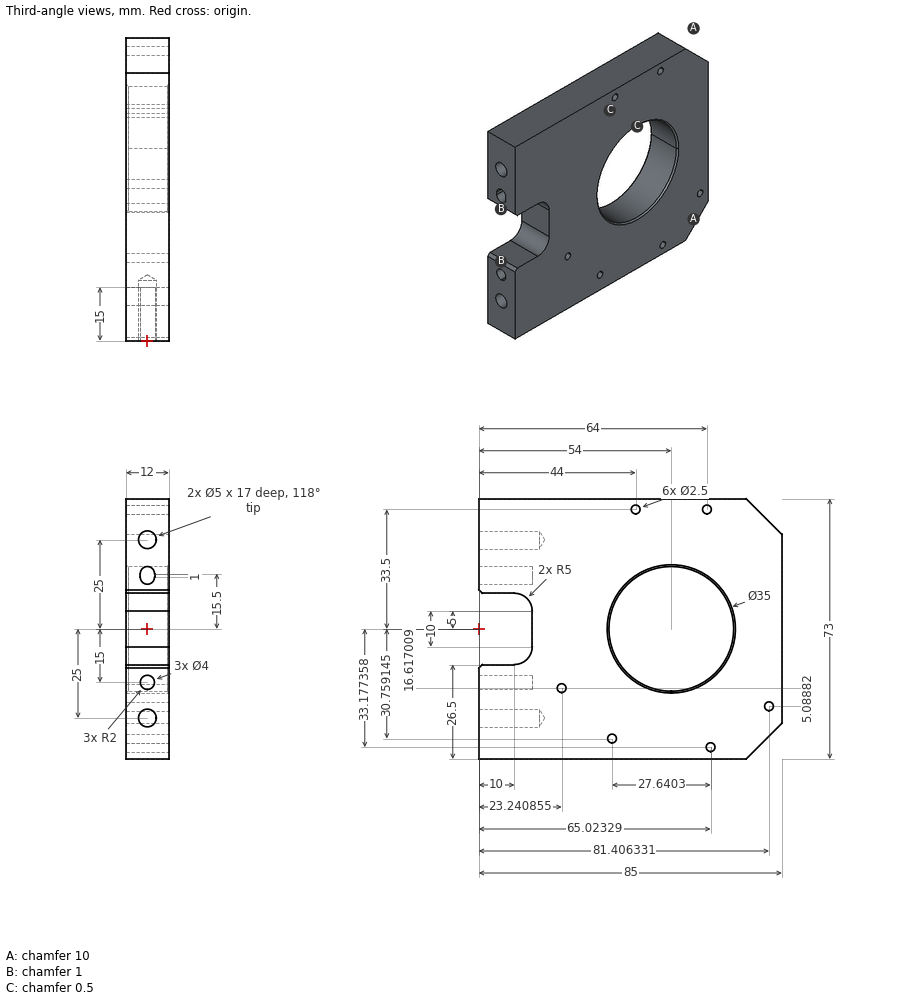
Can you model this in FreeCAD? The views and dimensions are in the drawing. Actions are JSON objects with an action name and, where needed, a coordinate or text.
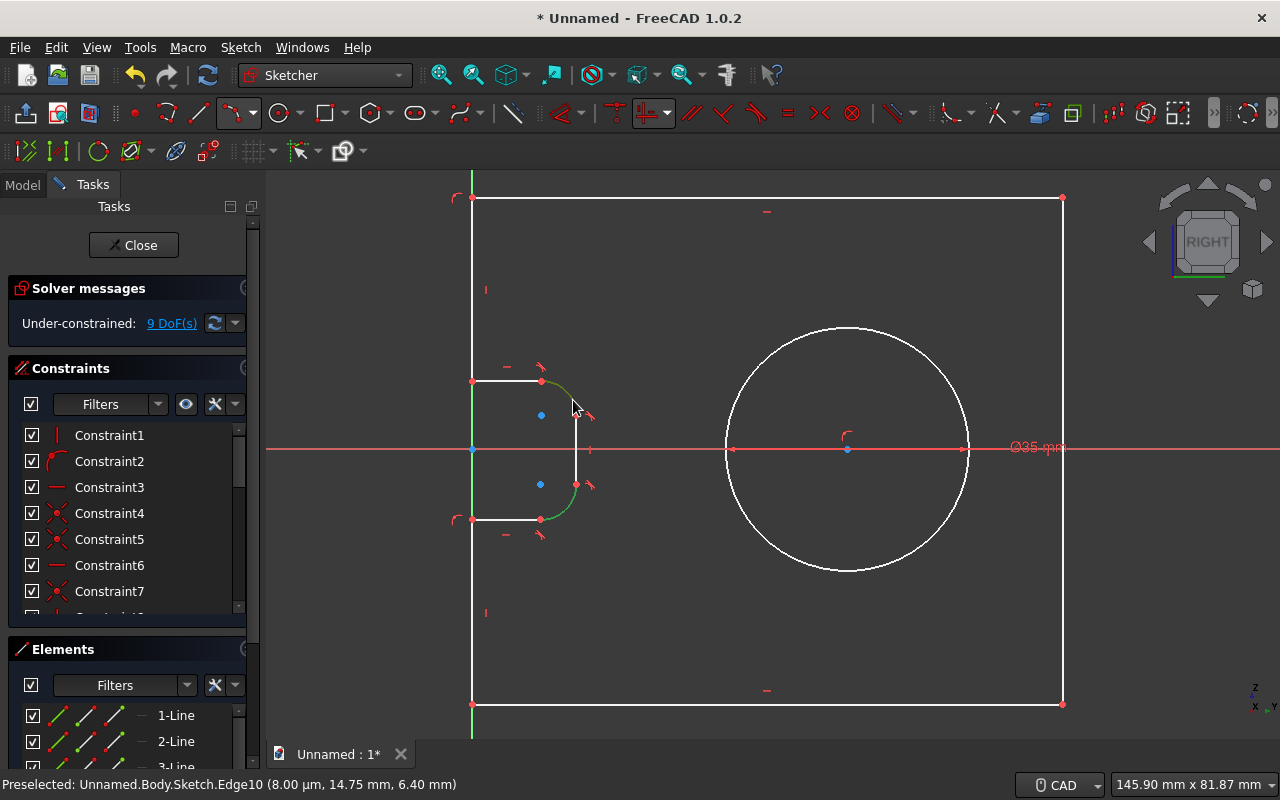
{"action": "left_click", "coordinate": [788, 114]}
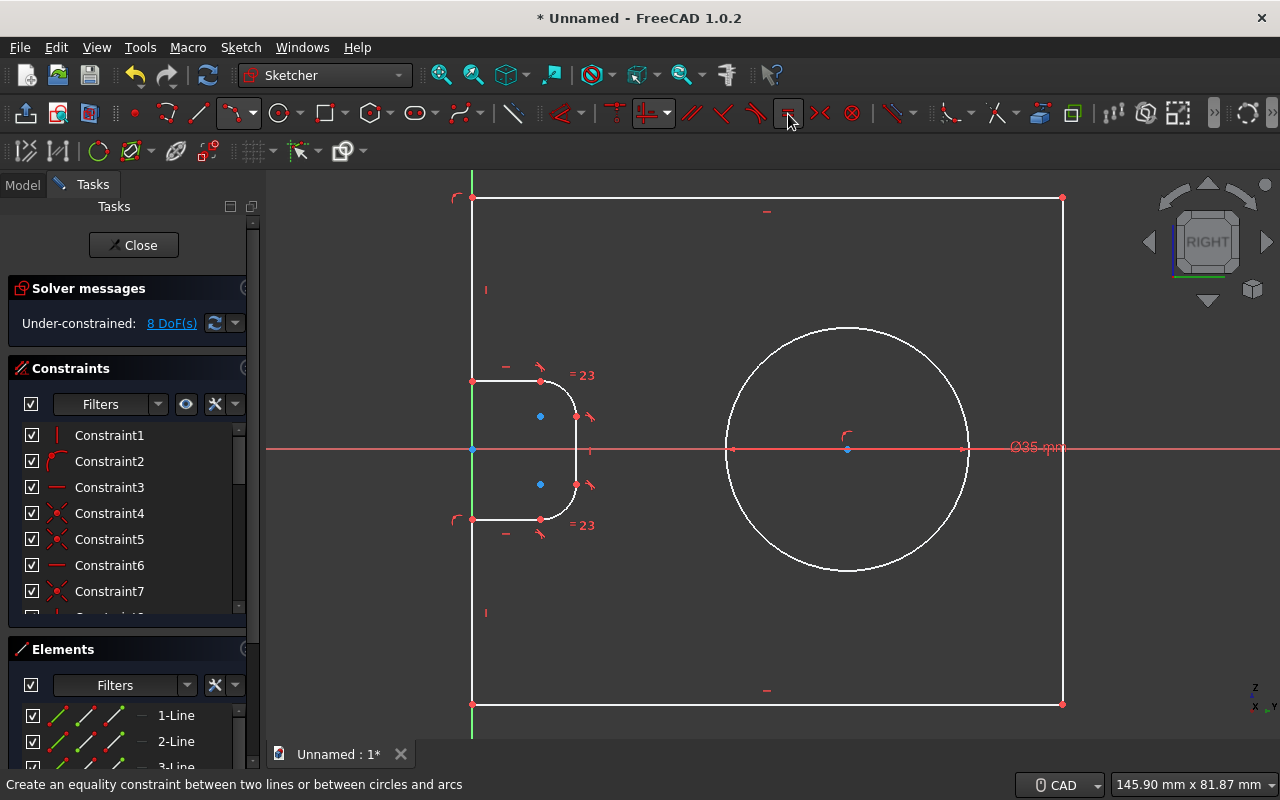
{"action": "left_click", "coordinate": [560, 114]}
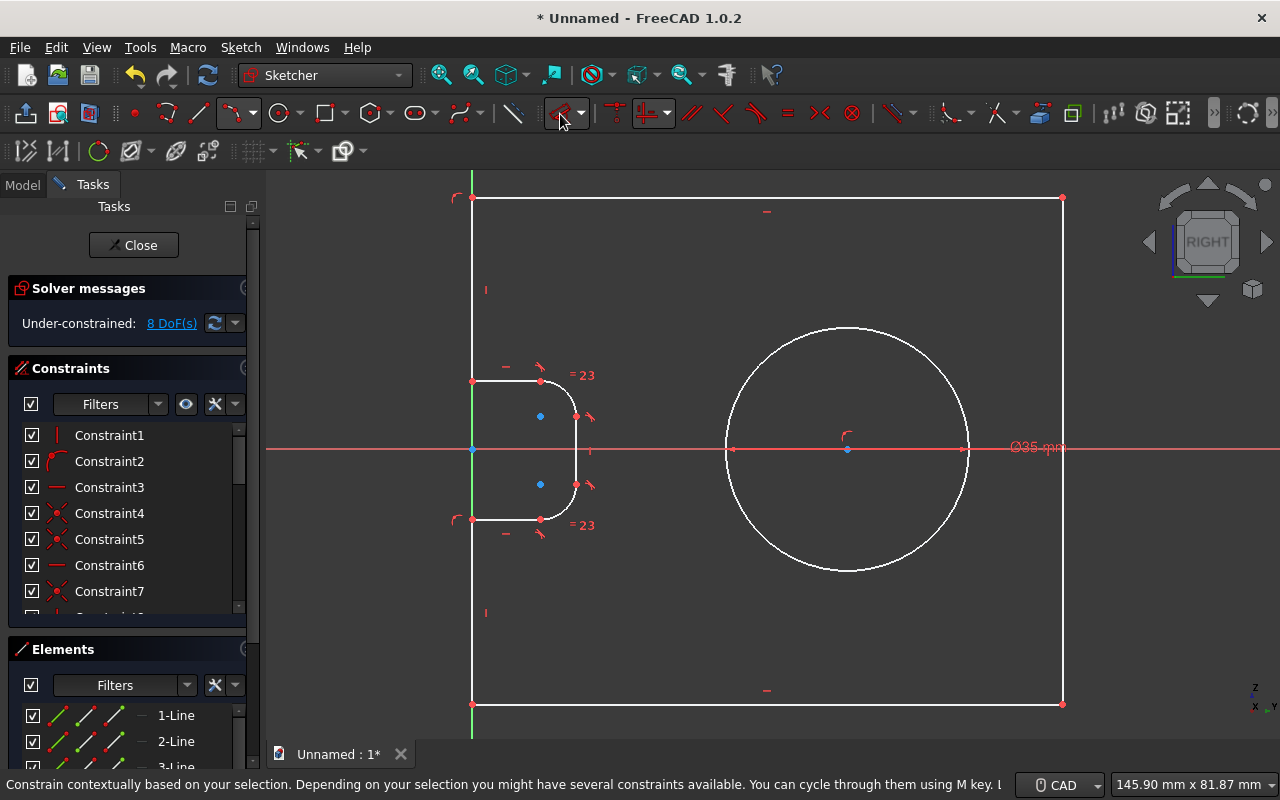
{"action": "left_click", "coordinate": [557, 516]}
{"action": "left_click", "coordinate": [572, 544]}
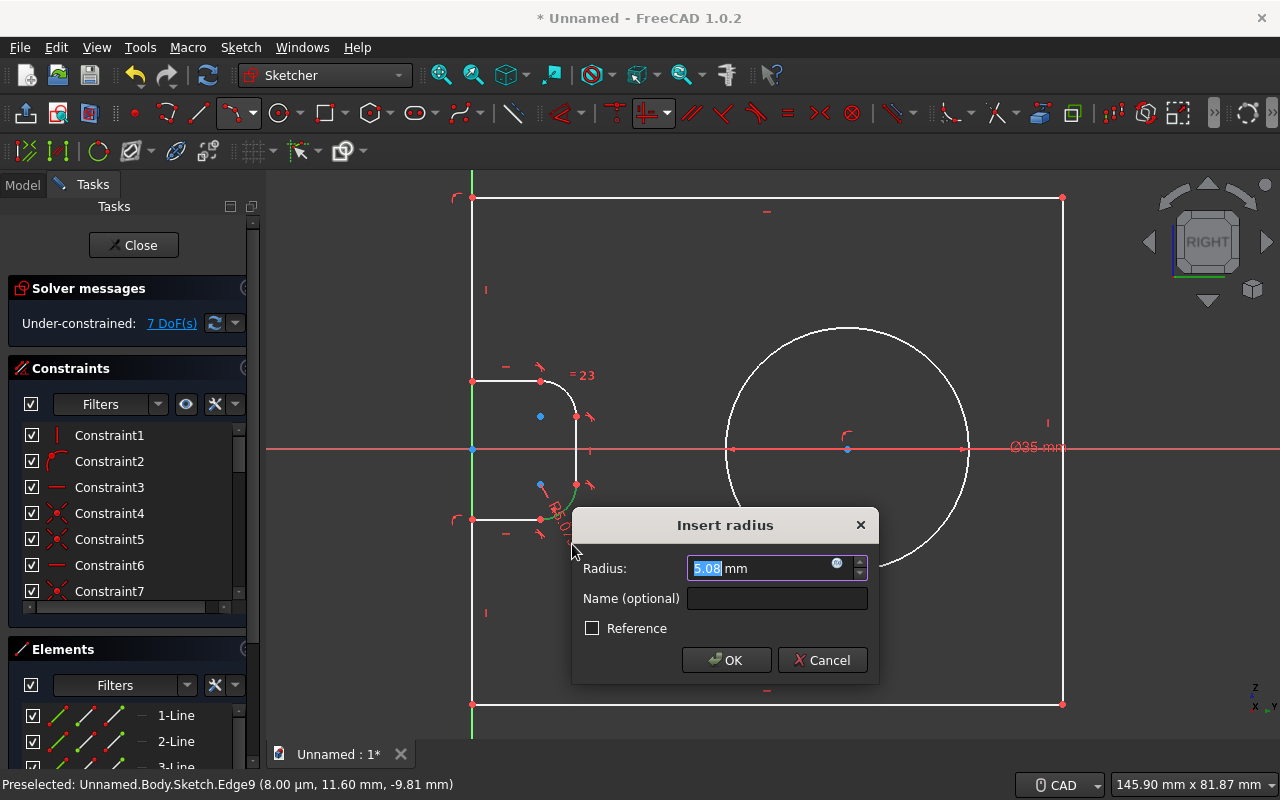
{"action": "type", "text": "5"}
{"action": "key", "text": "Return"}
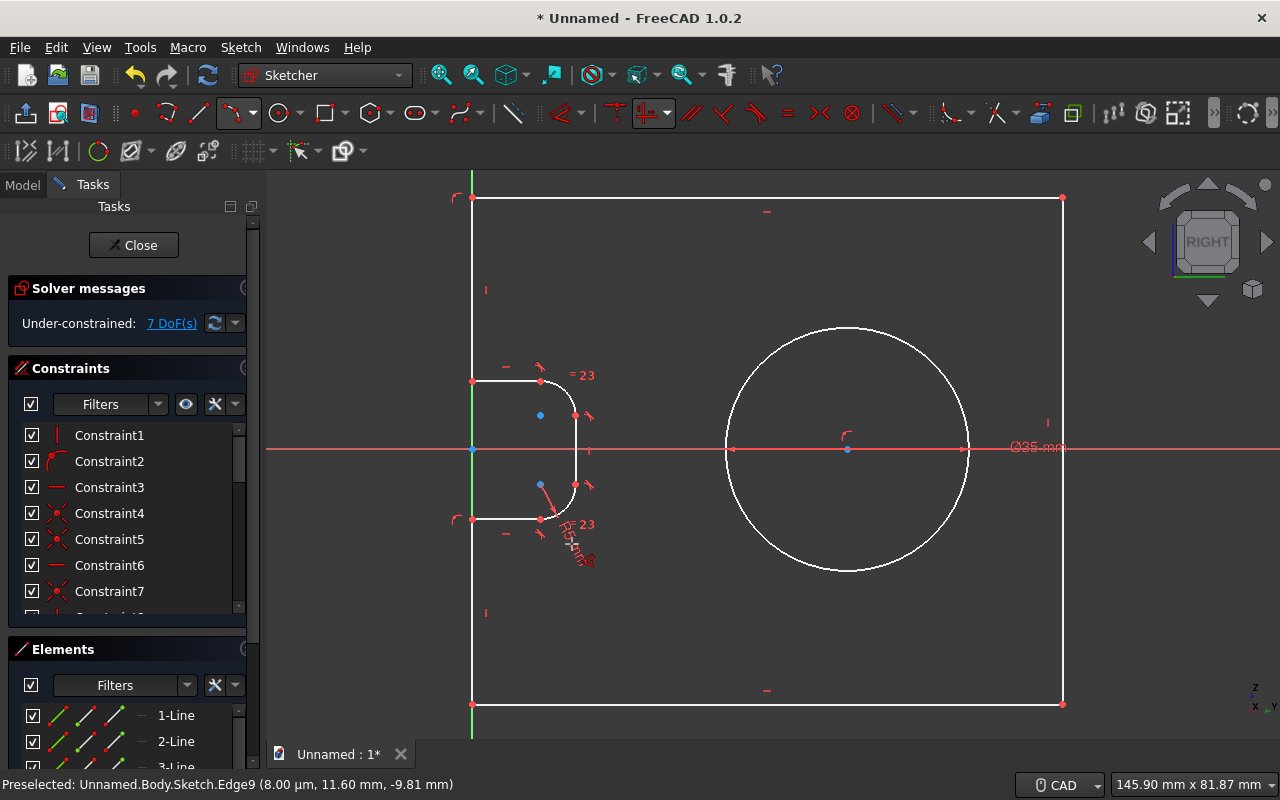
{"action": "left_click", "coordinate": [576, 436]}
{"action": "left_click", "coordinate": [542, 434]}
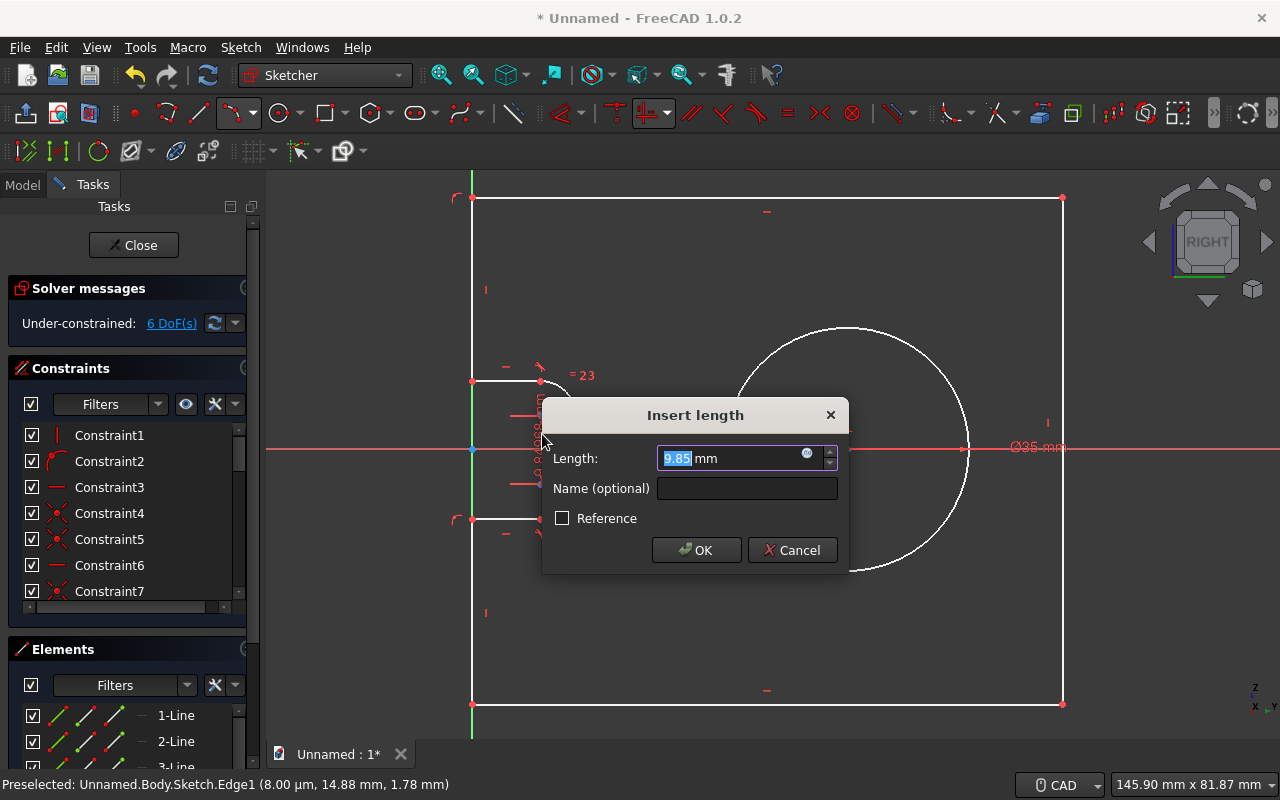
{"action": "type", "text": "10"}
{"action": "key", "text": "Return"}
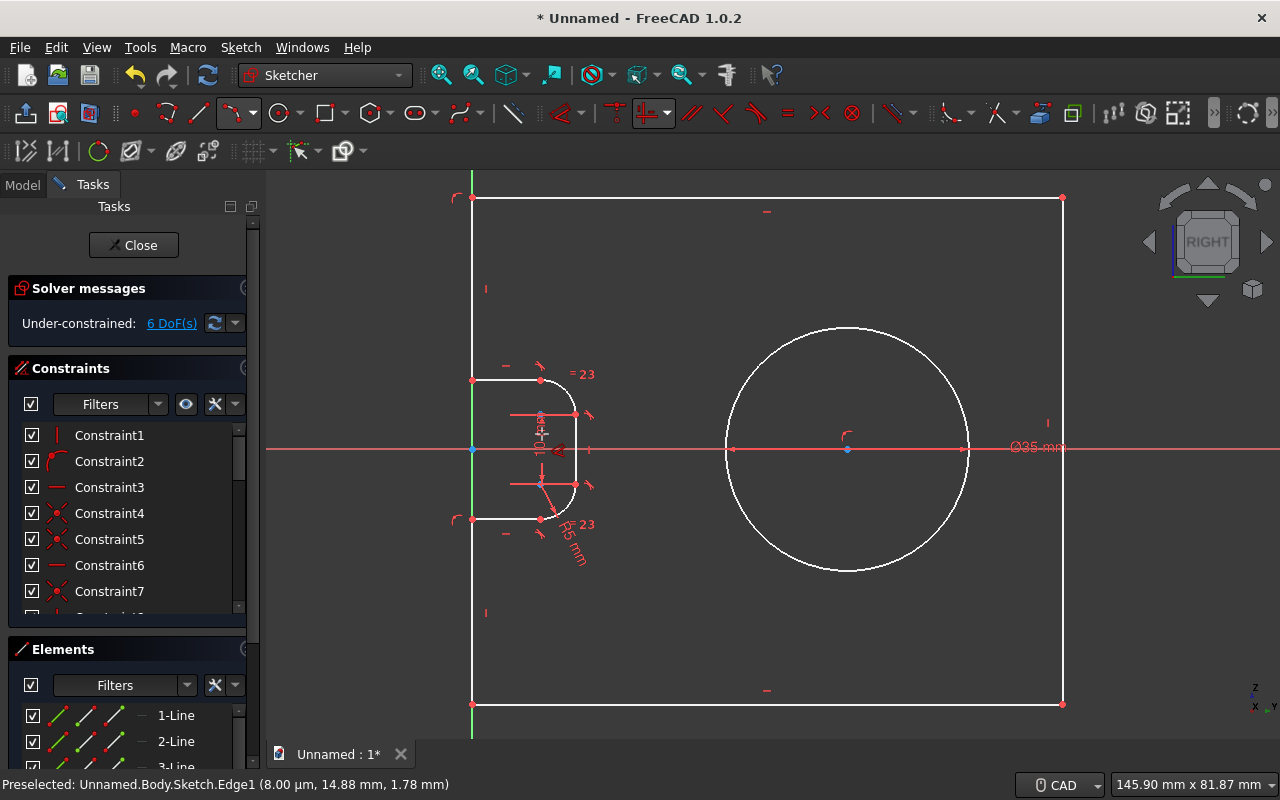
{"action": "left_click", "coordinate": [520, 519]}
{"action": "left_click", "coordinate": [491, 553]}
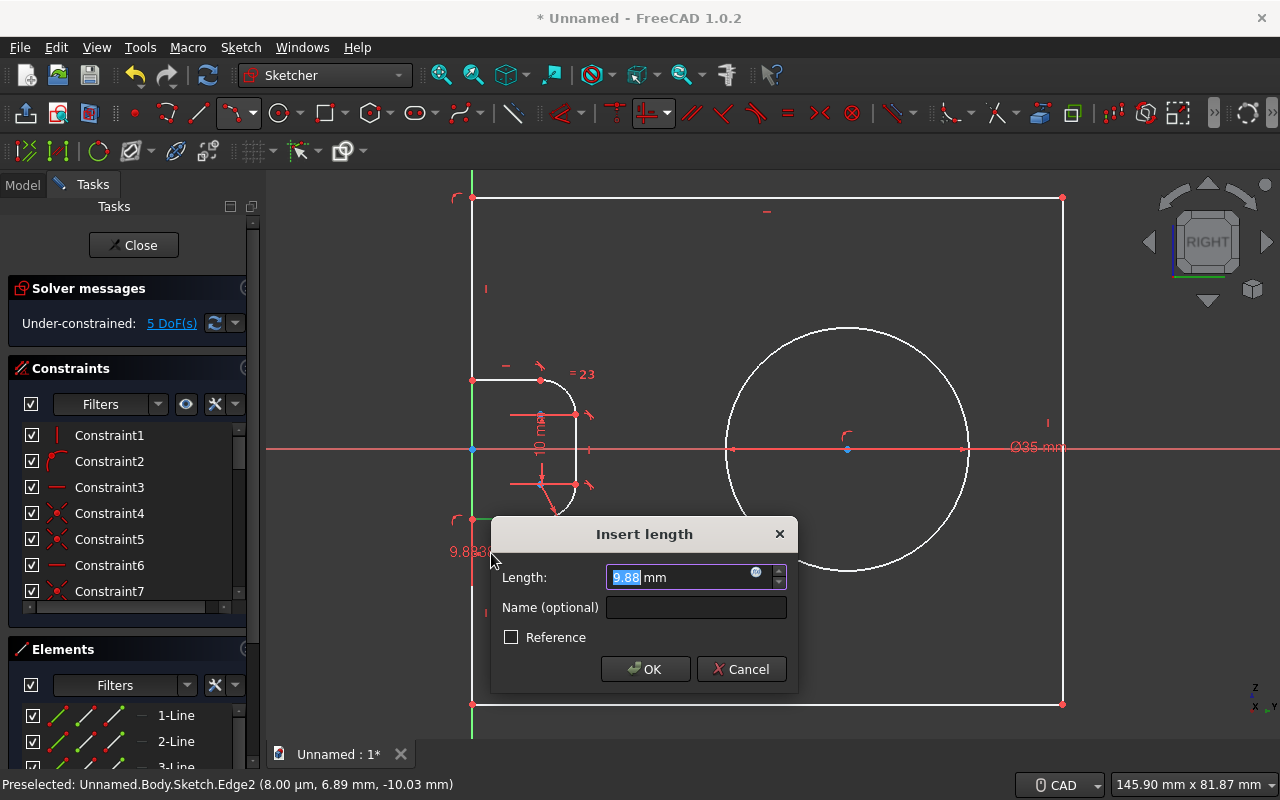
{"action": "type", "text": "10"}
{"action": "key", "text": "Return"}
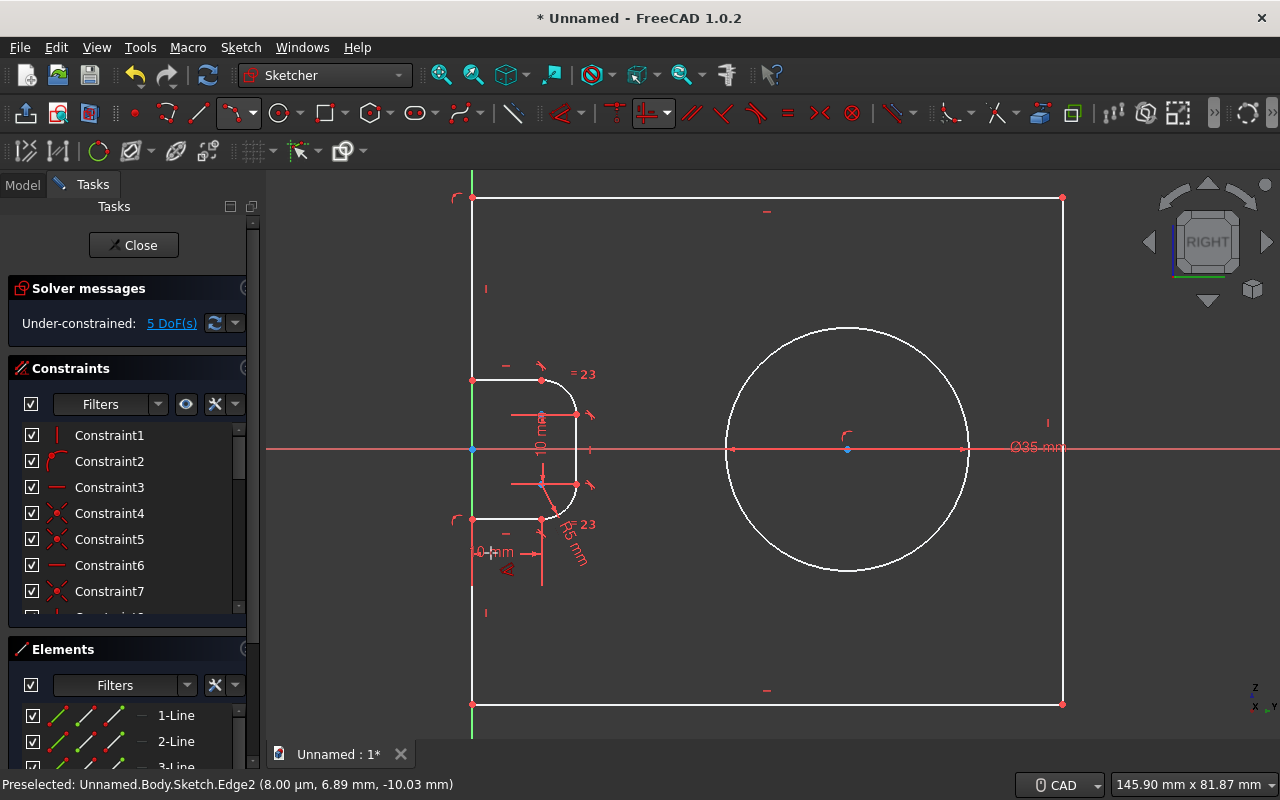
{"action": "left_click", "coordinate": [649, 705]}
{"action": "left_click", "coordinate": [767, 671]}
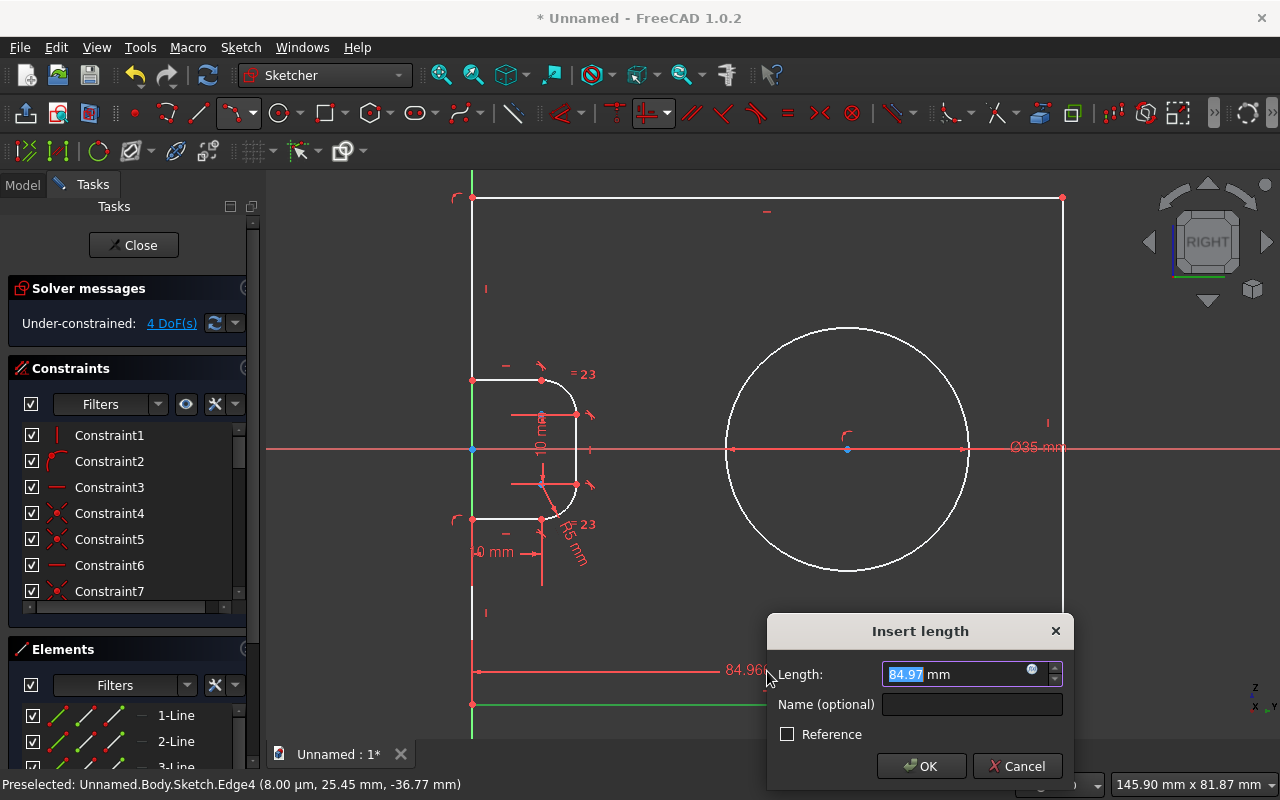
{"action": "type", "text": "85"}
{"action": "key", "text": "Return"}